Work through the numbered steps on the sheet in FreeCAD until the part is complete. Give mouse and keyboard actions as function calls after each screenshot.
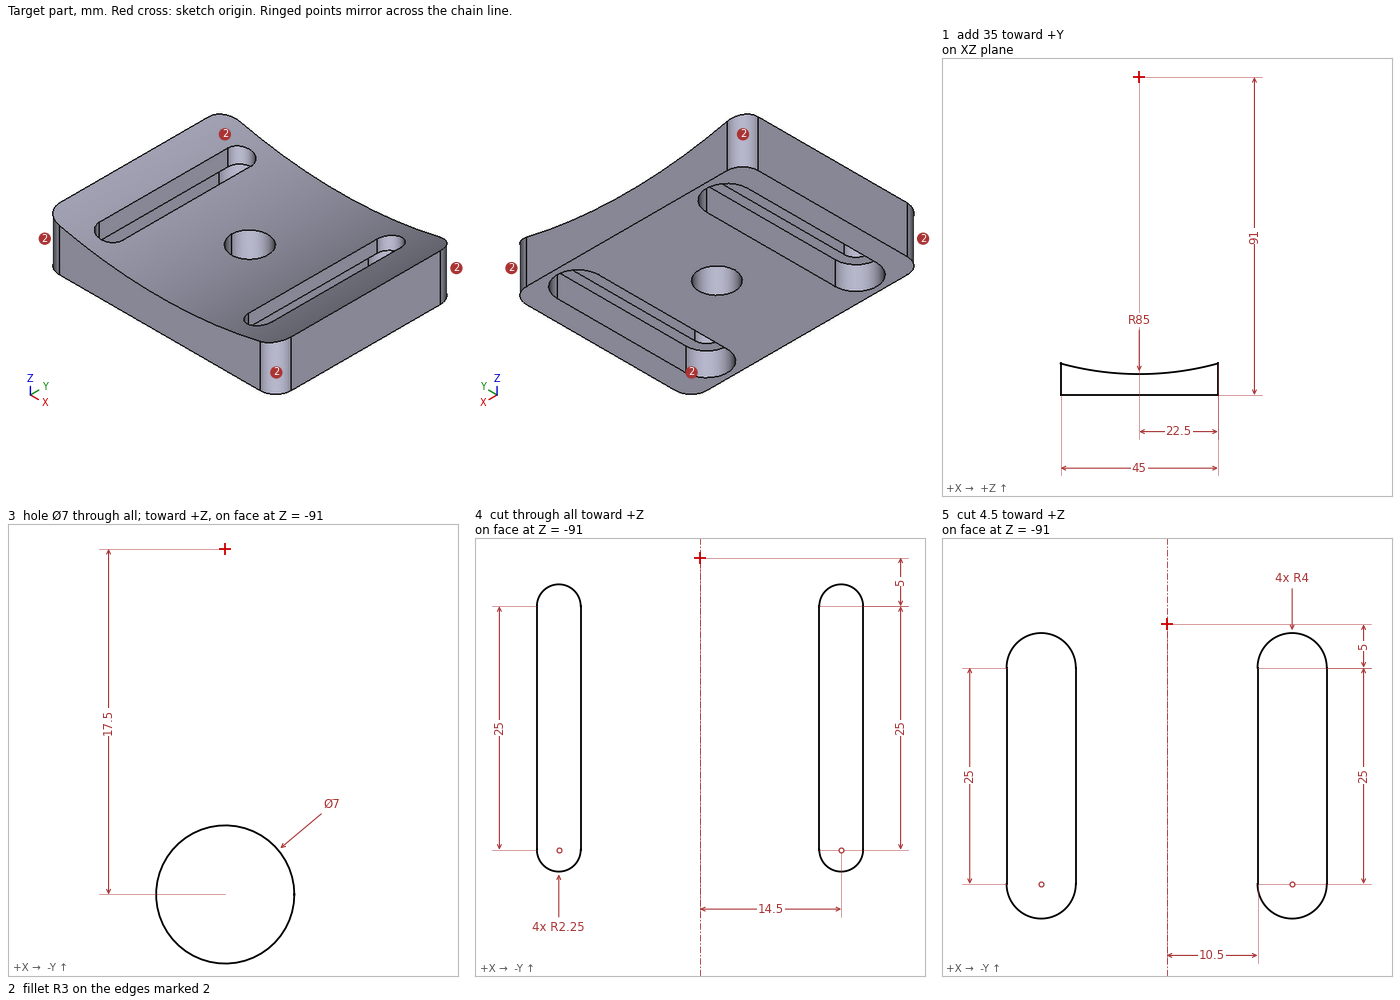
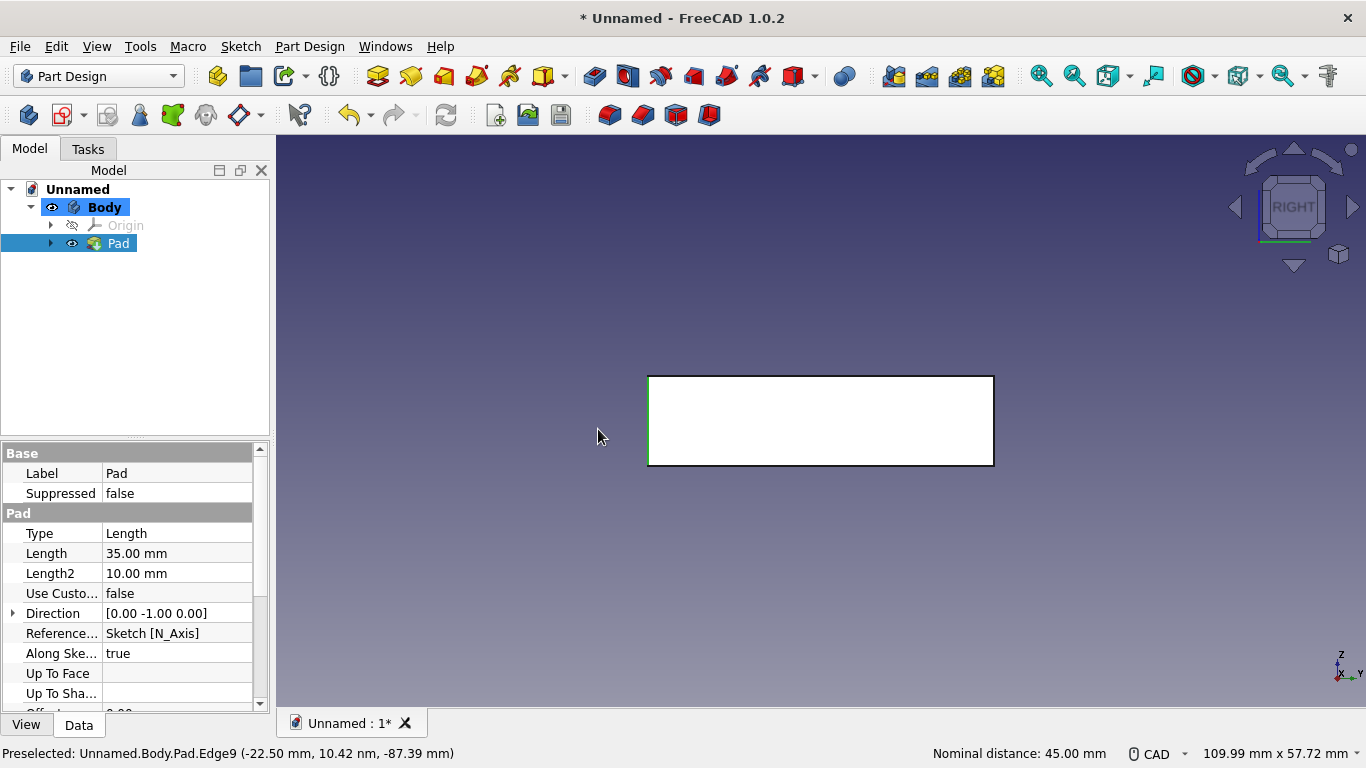
click(1042, 76)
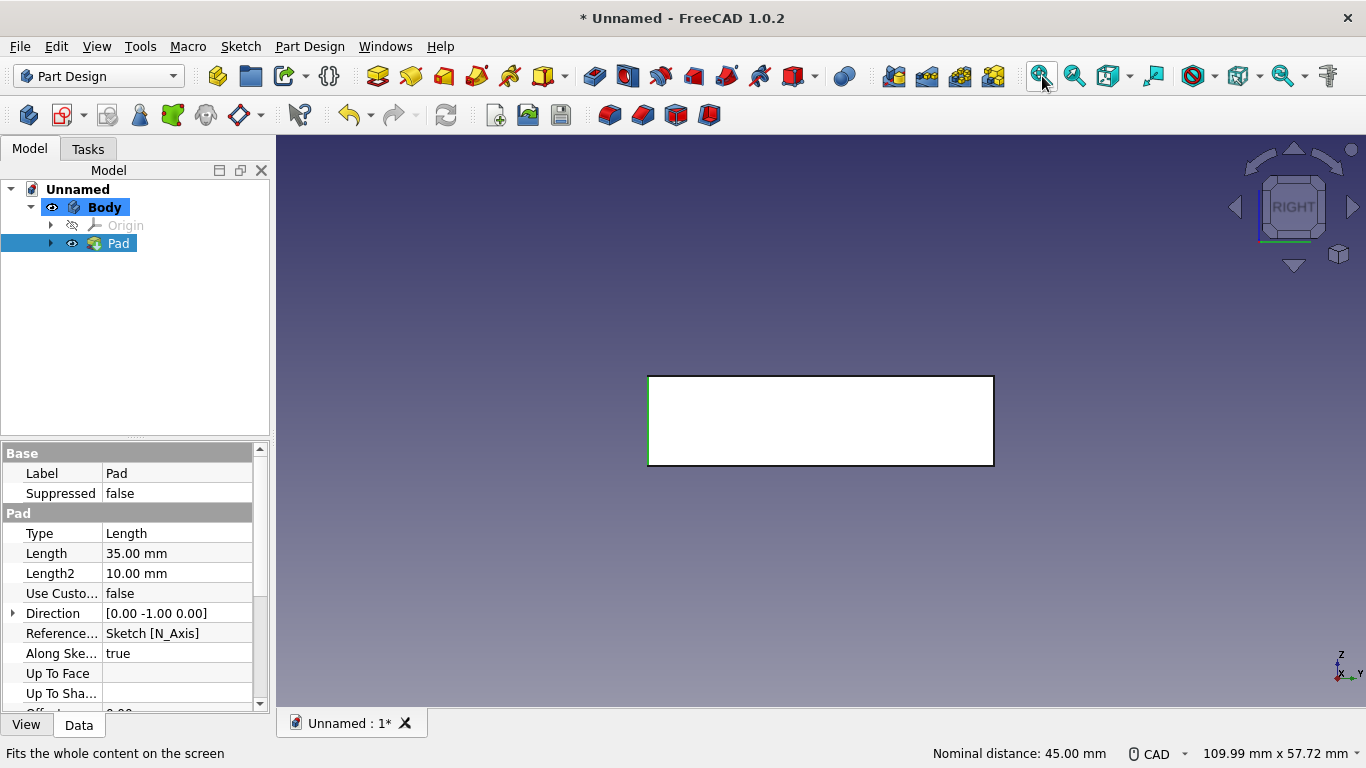
click(994, 420, ctrl)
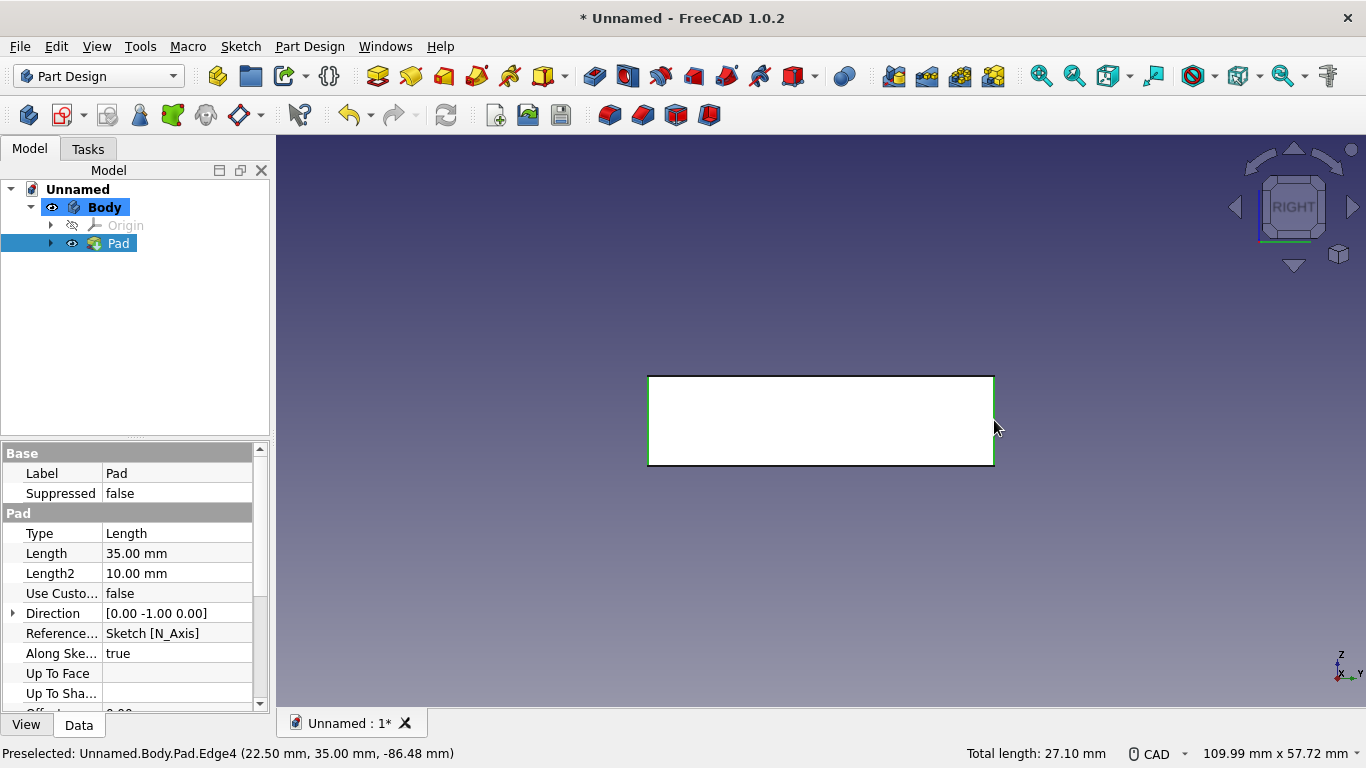
key(5)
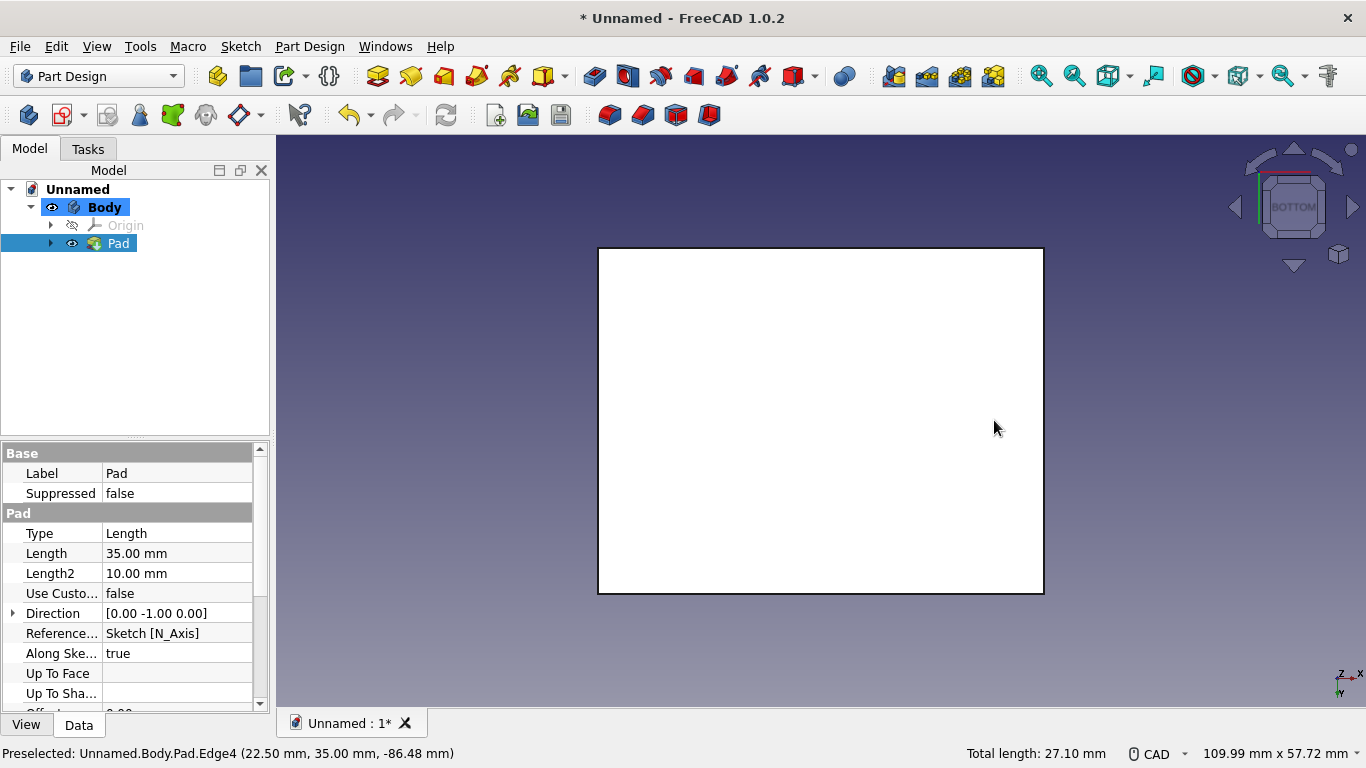
key(4)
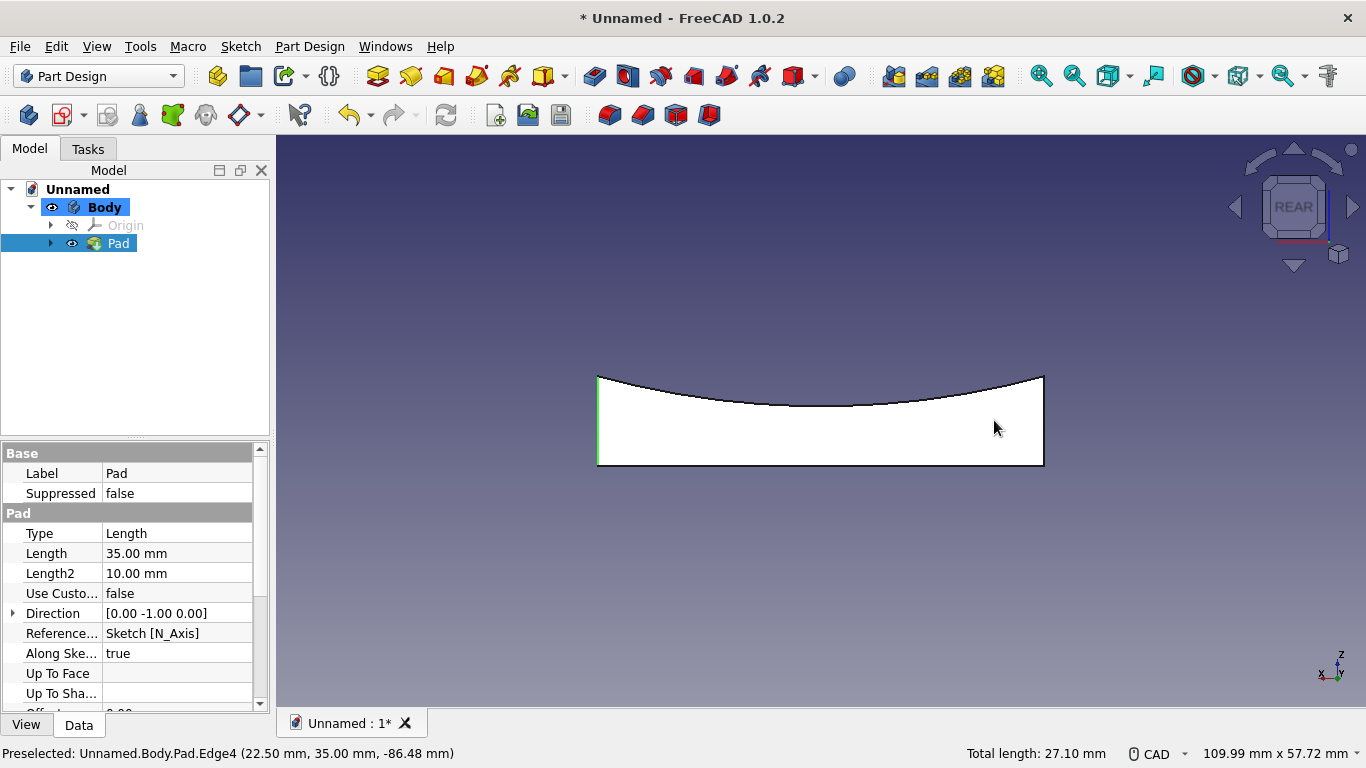
key(v)
key(f)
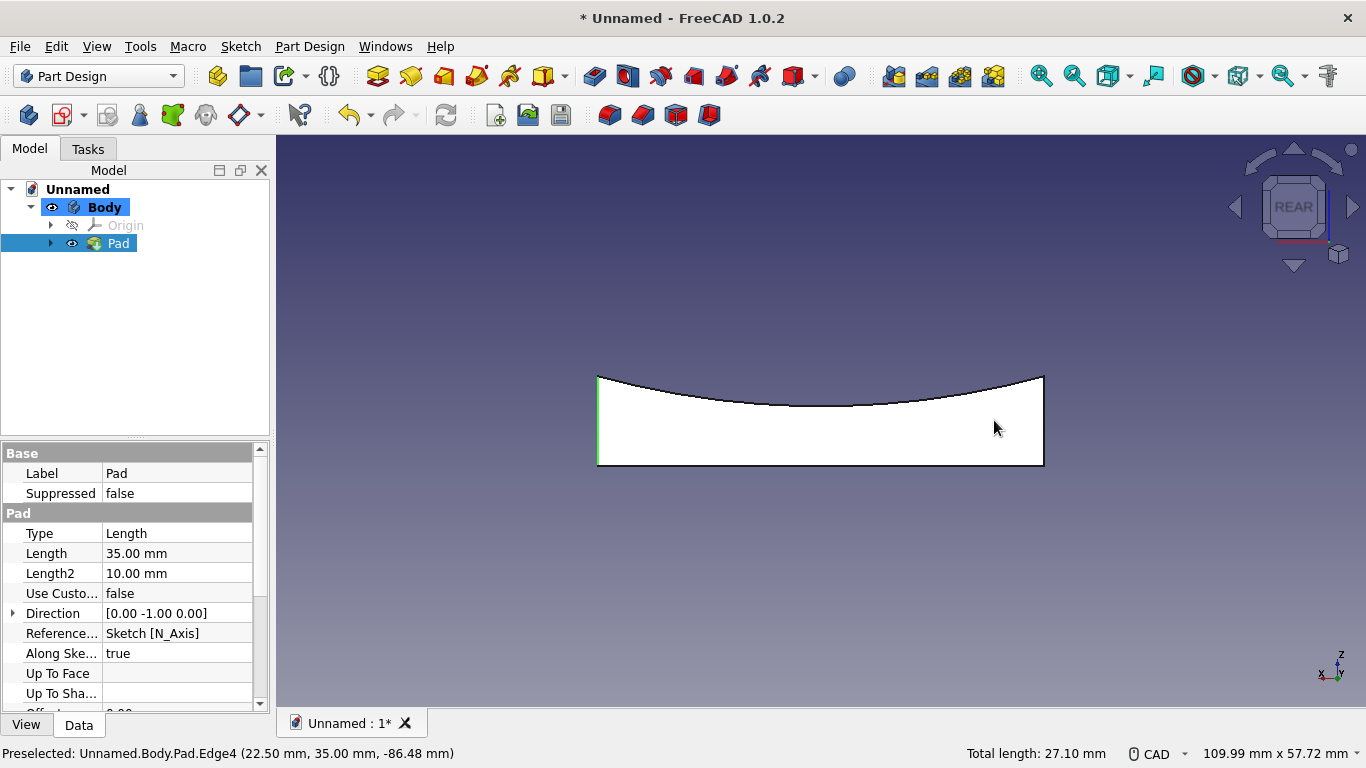
click(1044, 420, ctrl)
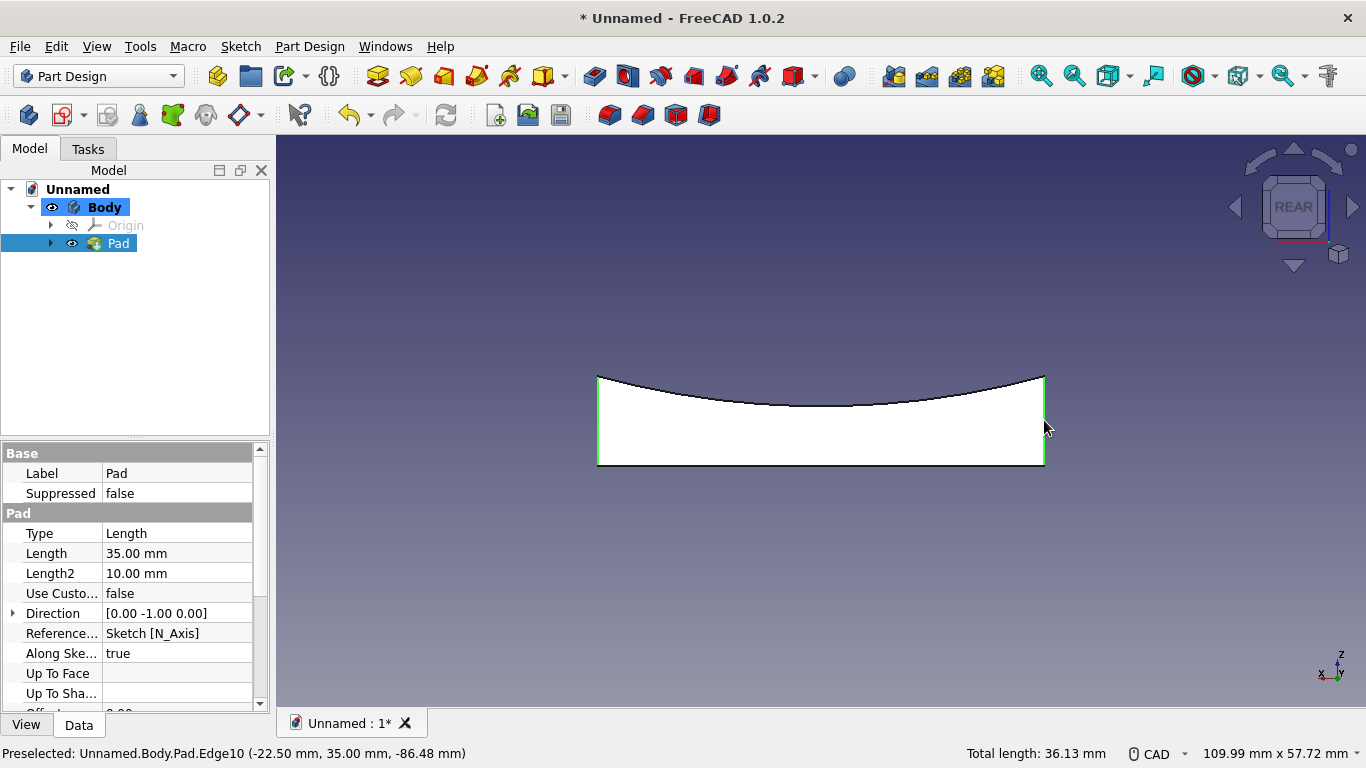
click(610, 116)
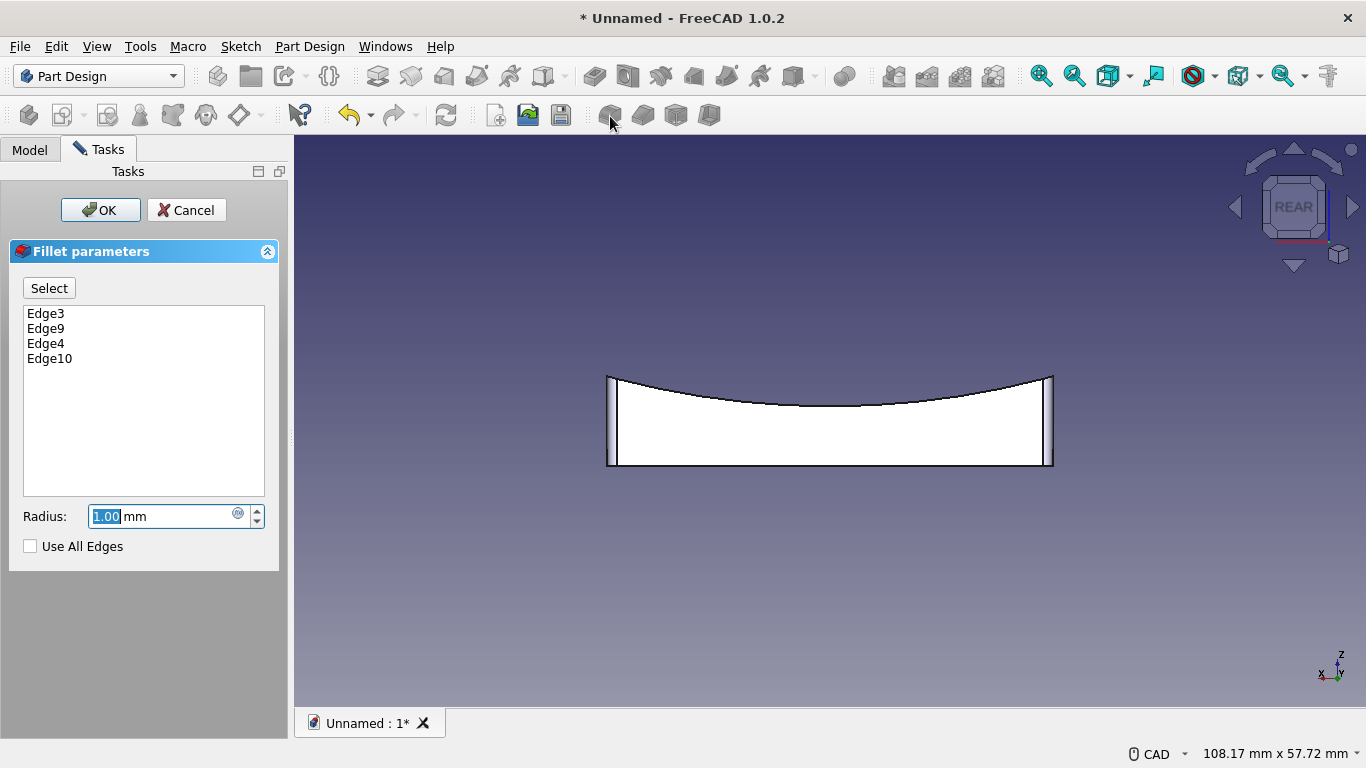
text(3)
key(Tab)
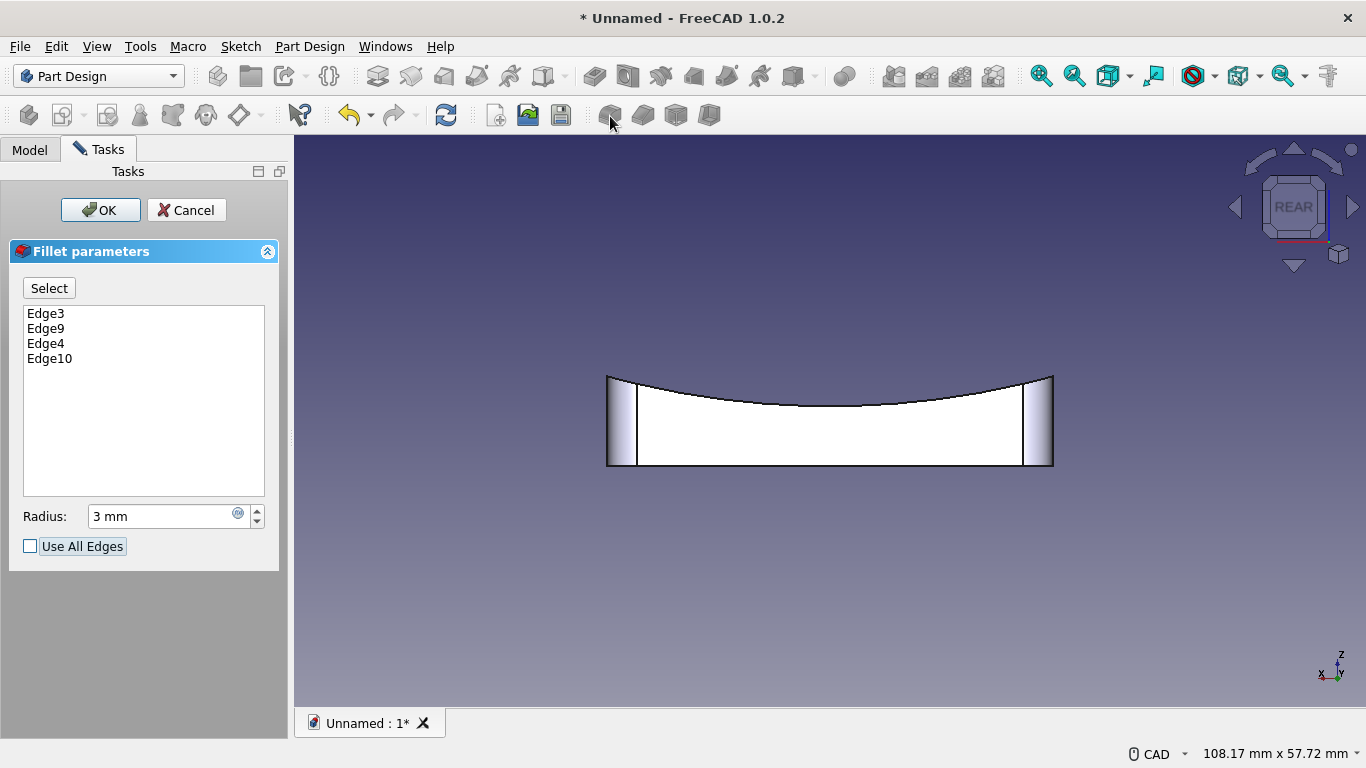
click(101, 210)